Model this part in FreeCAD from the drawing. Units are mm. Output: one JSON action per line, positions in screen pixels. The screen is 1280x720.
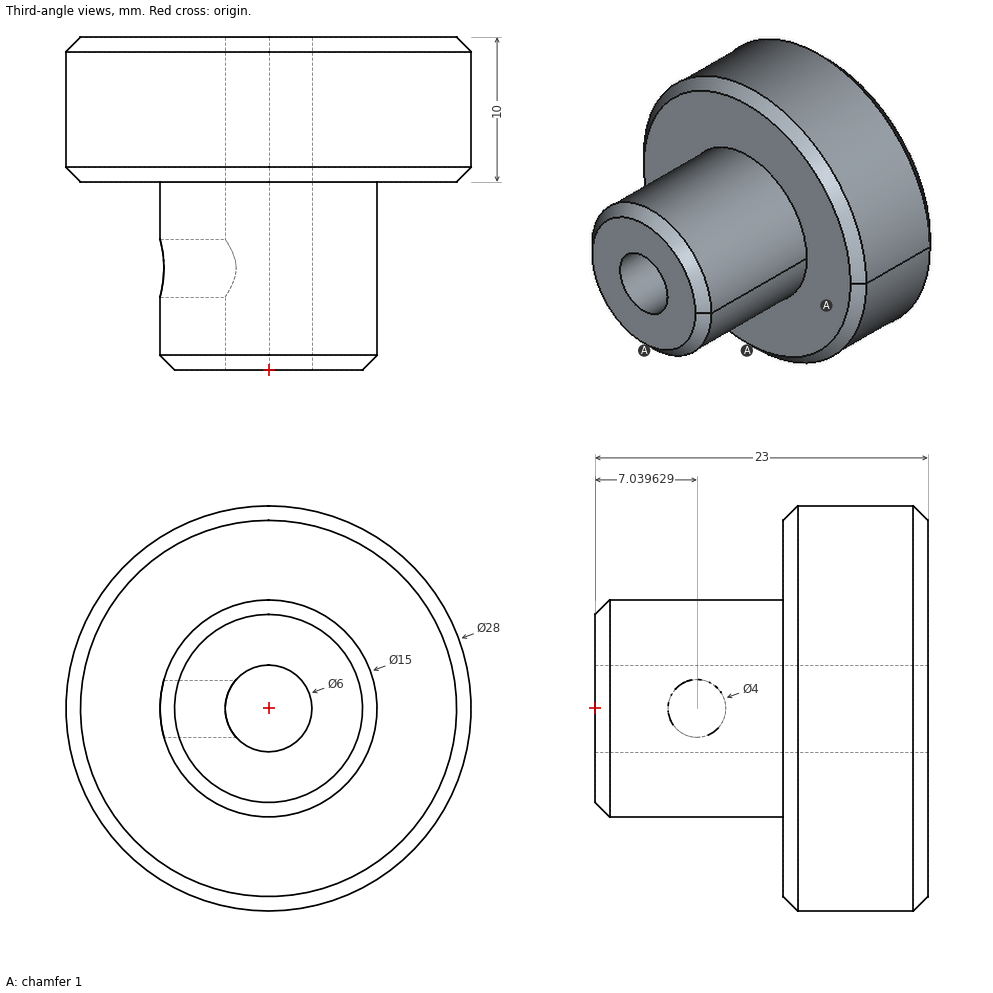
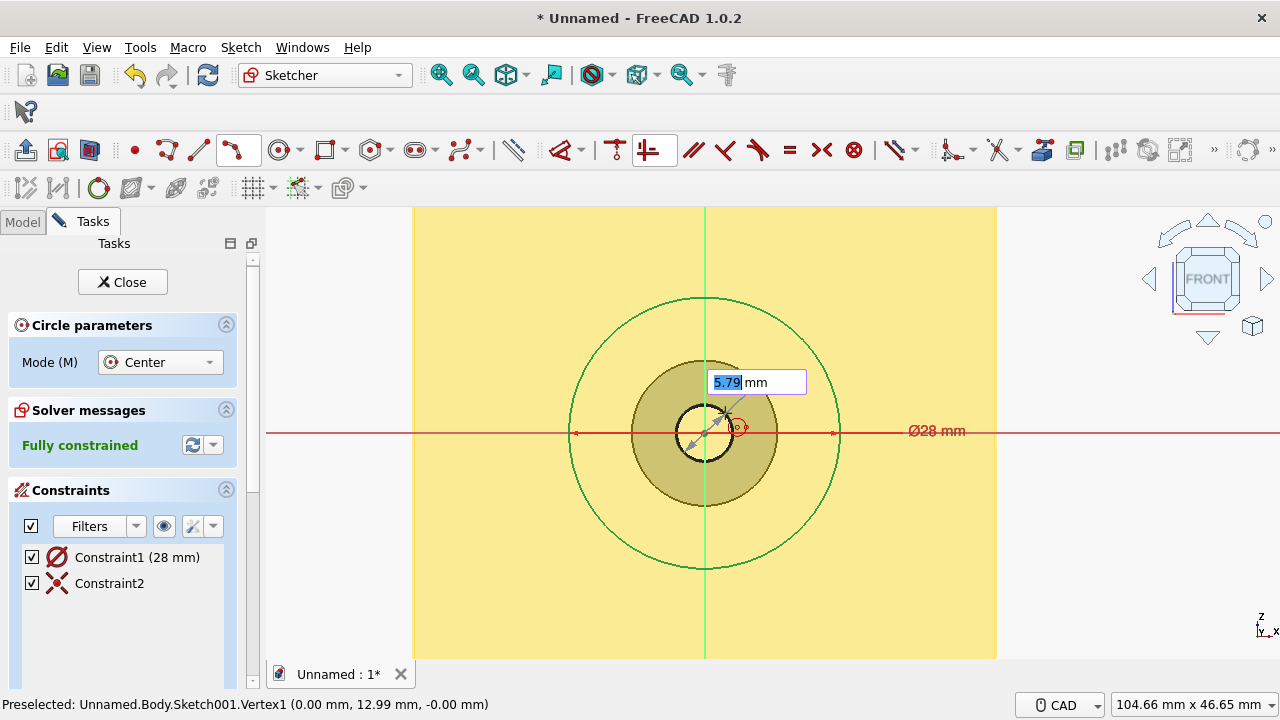
{"action": "type", "text": "6"}
{"action": "key", "text": "Return"}
{"action": "key", "text": "Escape"}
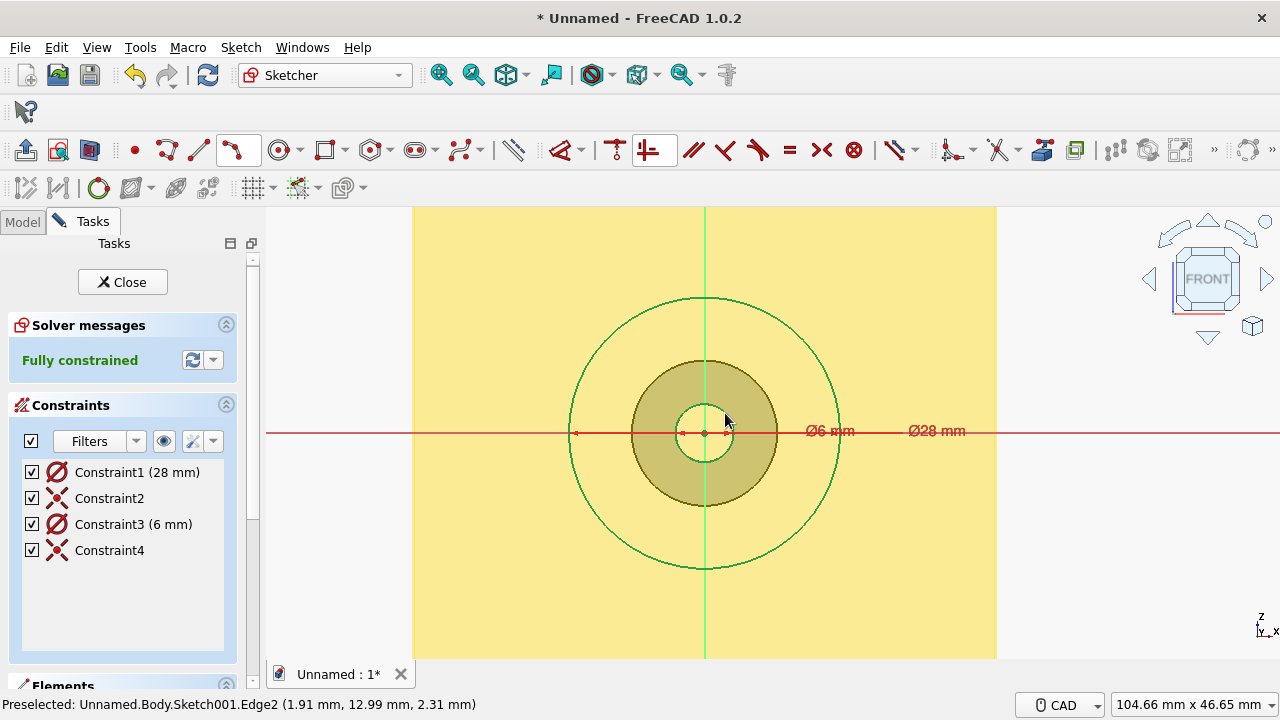
{"action": "left_click", "coordinate": [123, 282]}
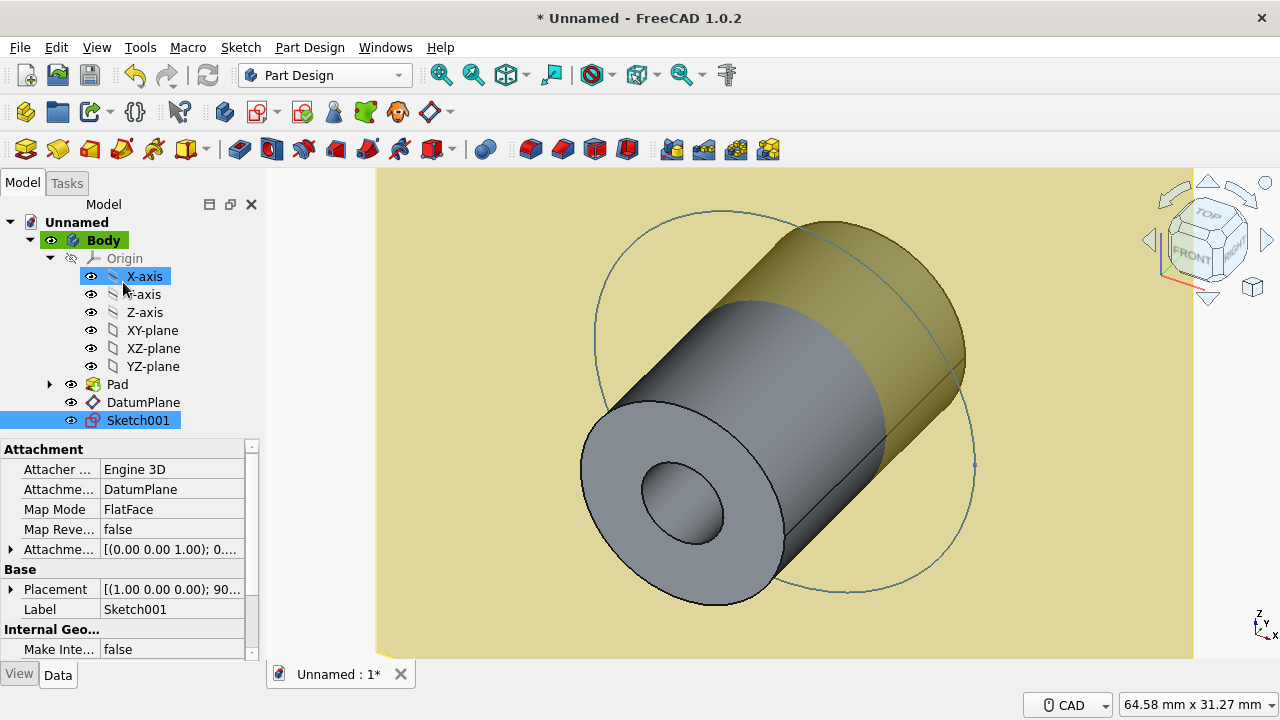
{"action": "left_click", "coordinate": [26, 150]}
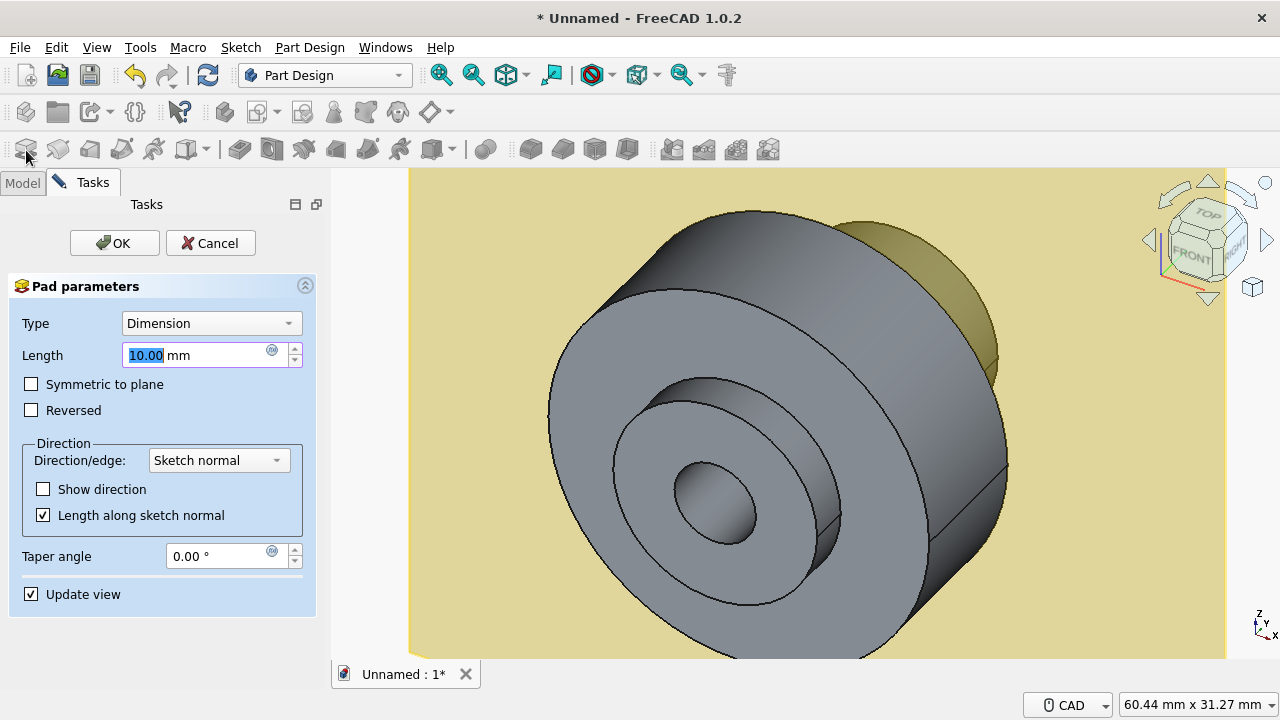
{"action": "type", "text": "10"}
{"action": "key", "text": "Tab"}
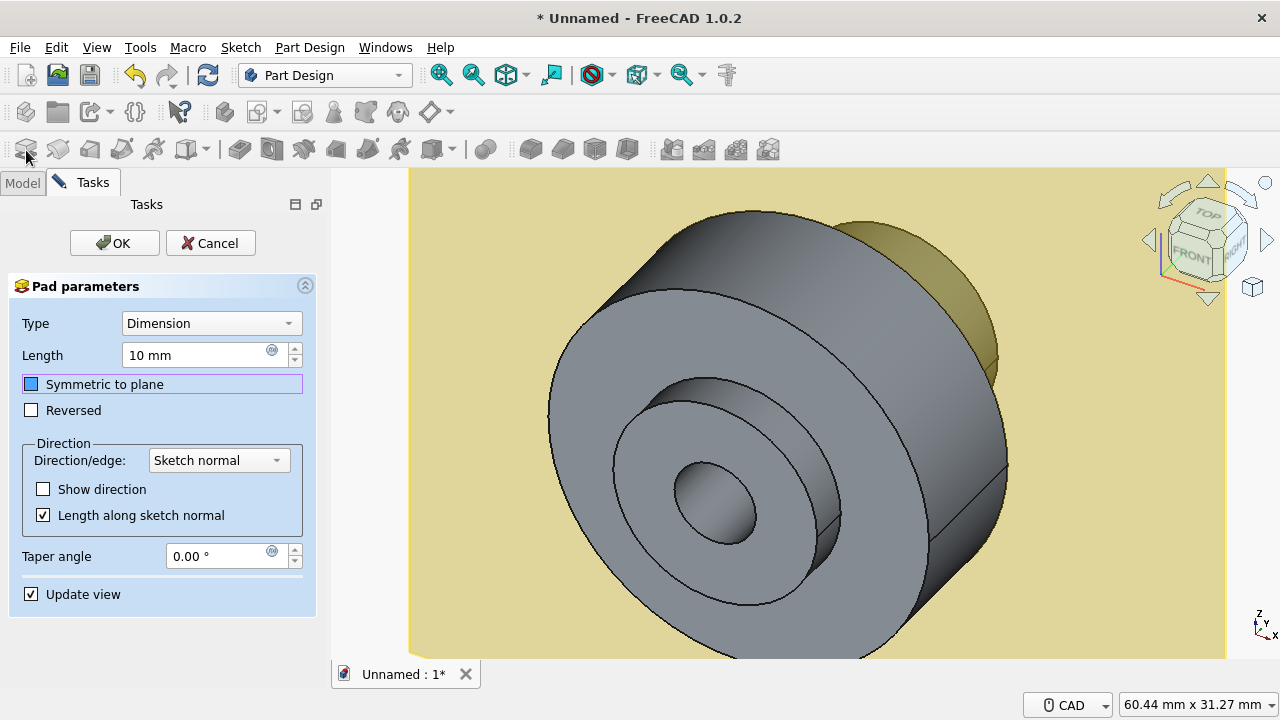
{"action": "left_click", "coordinate": [30, 410]}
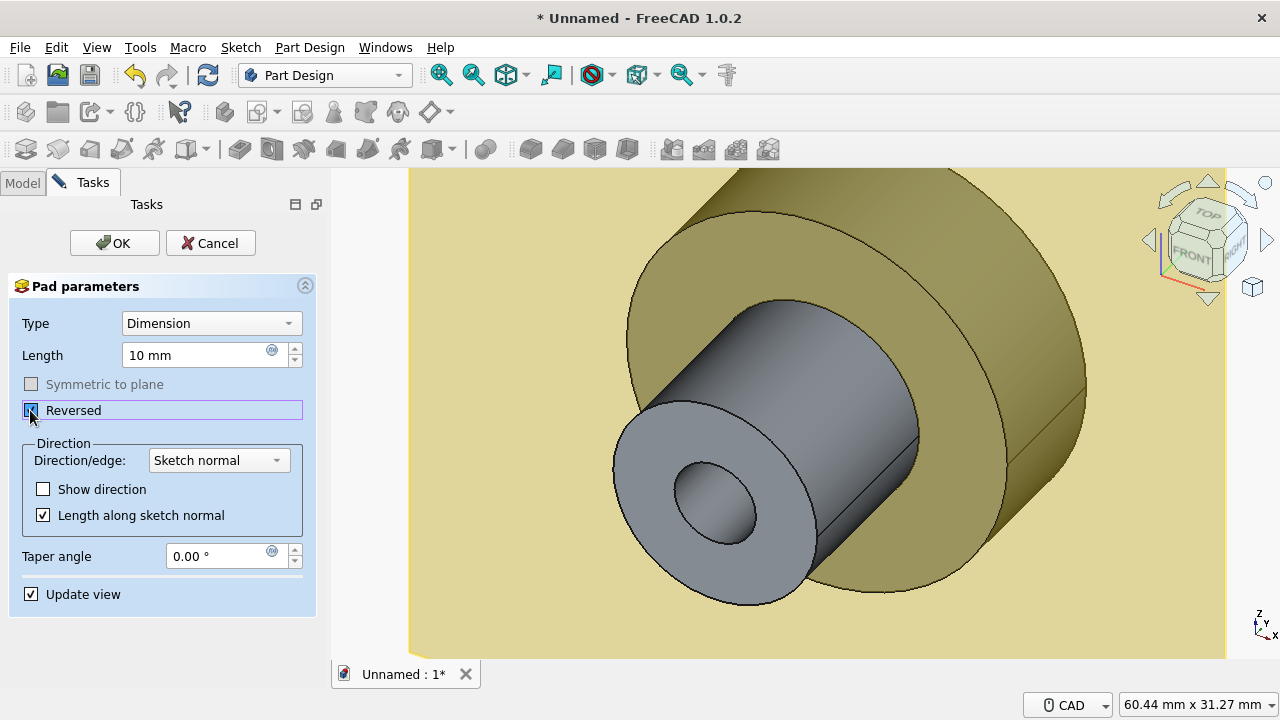
{"action": "left_click", "coordinate": [115, 243]}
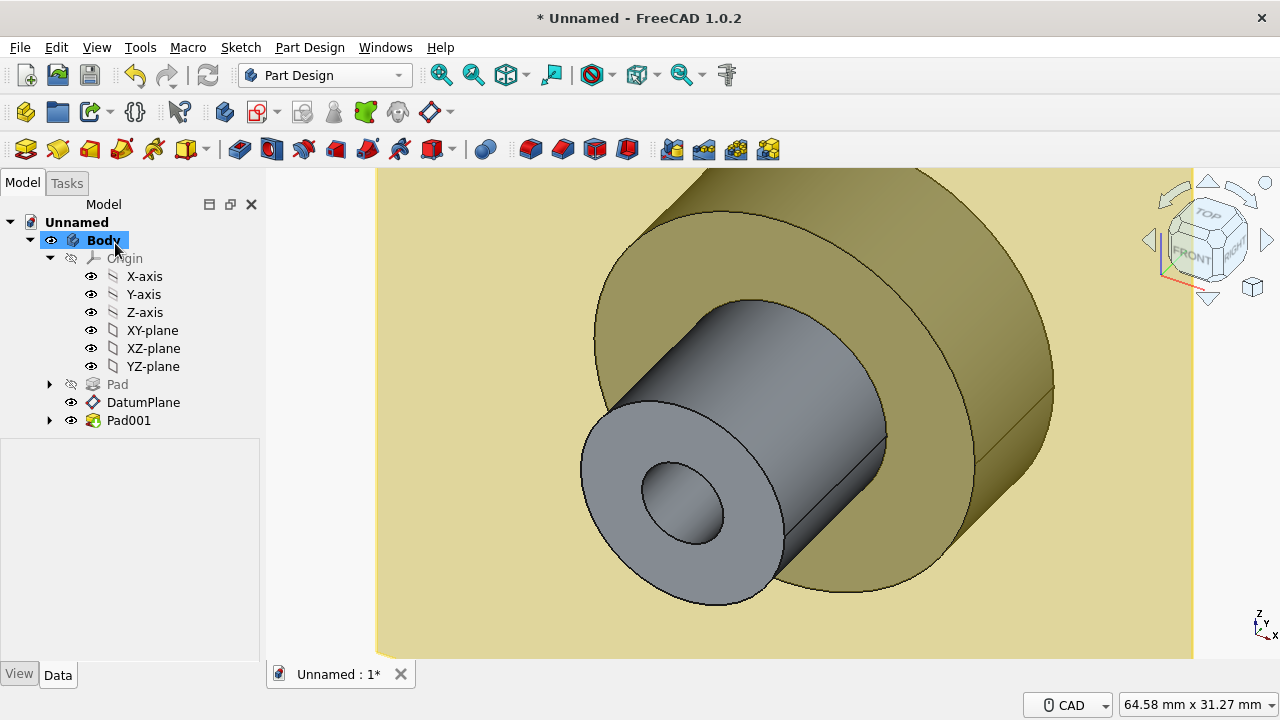
{"action": "left_click", "coordinate": [116, 402]}
{"action": "key", "text": "space"}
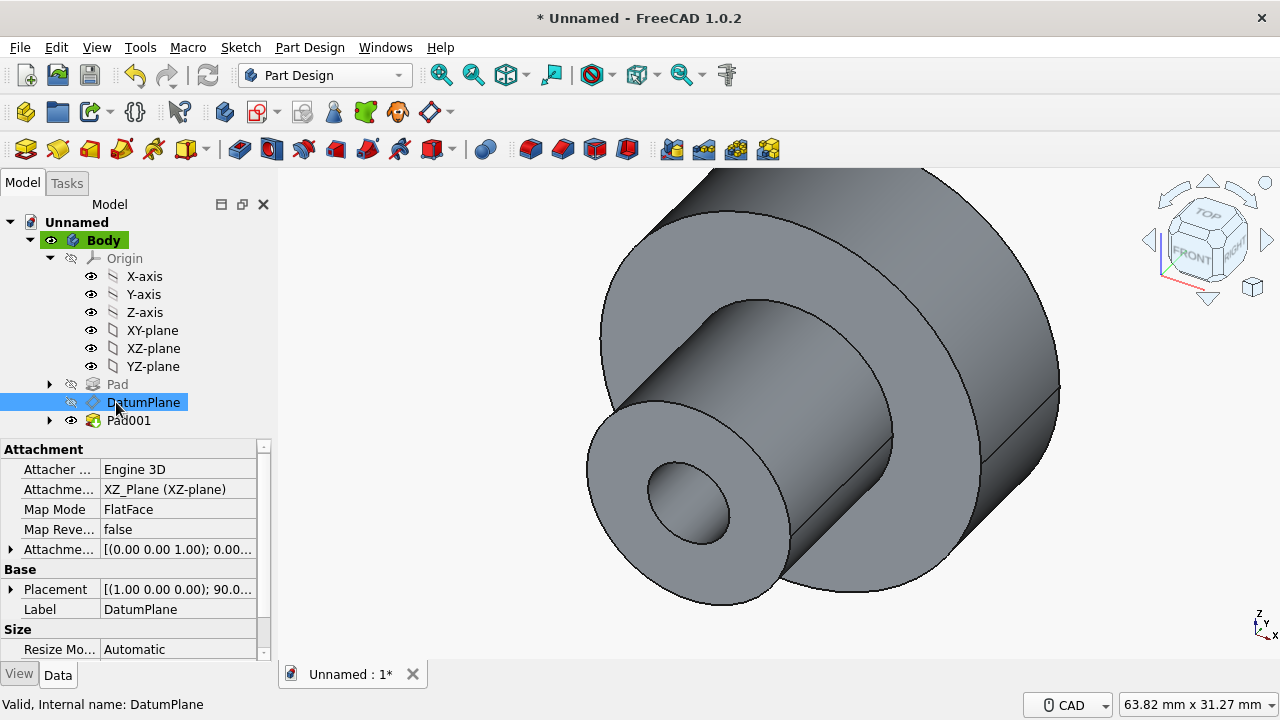
{"action": "left_click", "coordinate": [442, 76]}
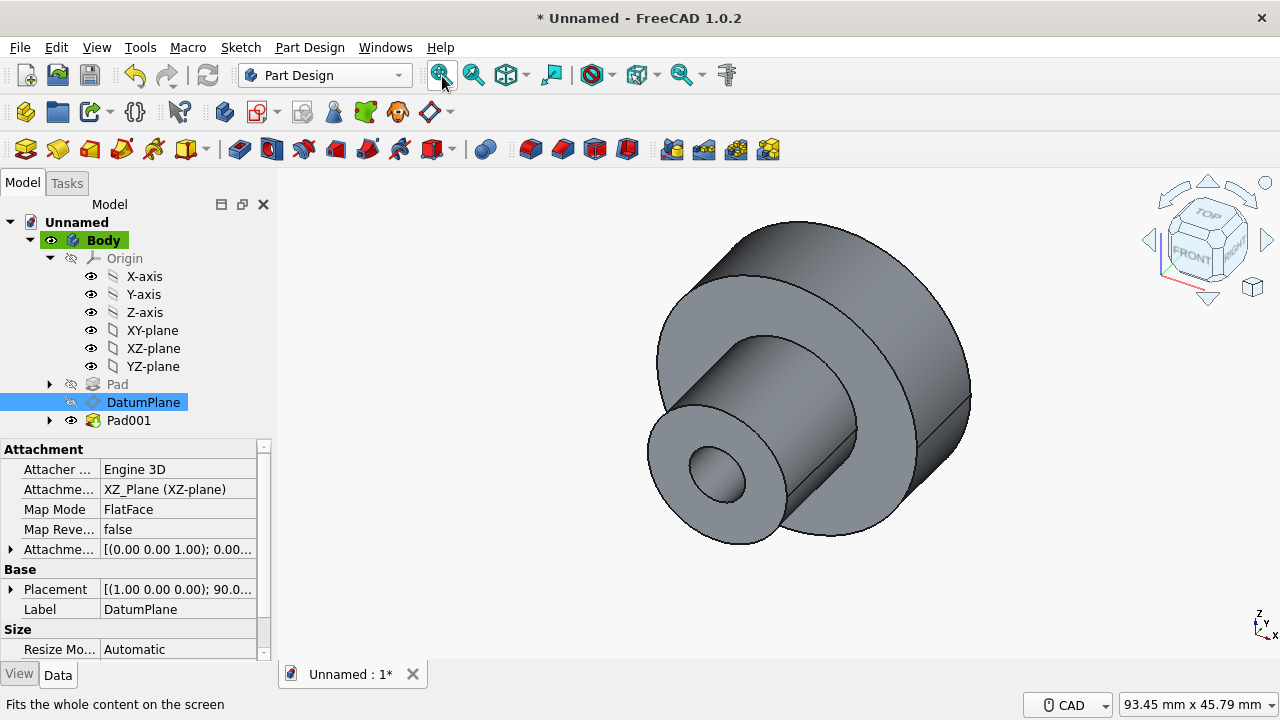
{"action": "left_click", "coordinate": [682, 297]}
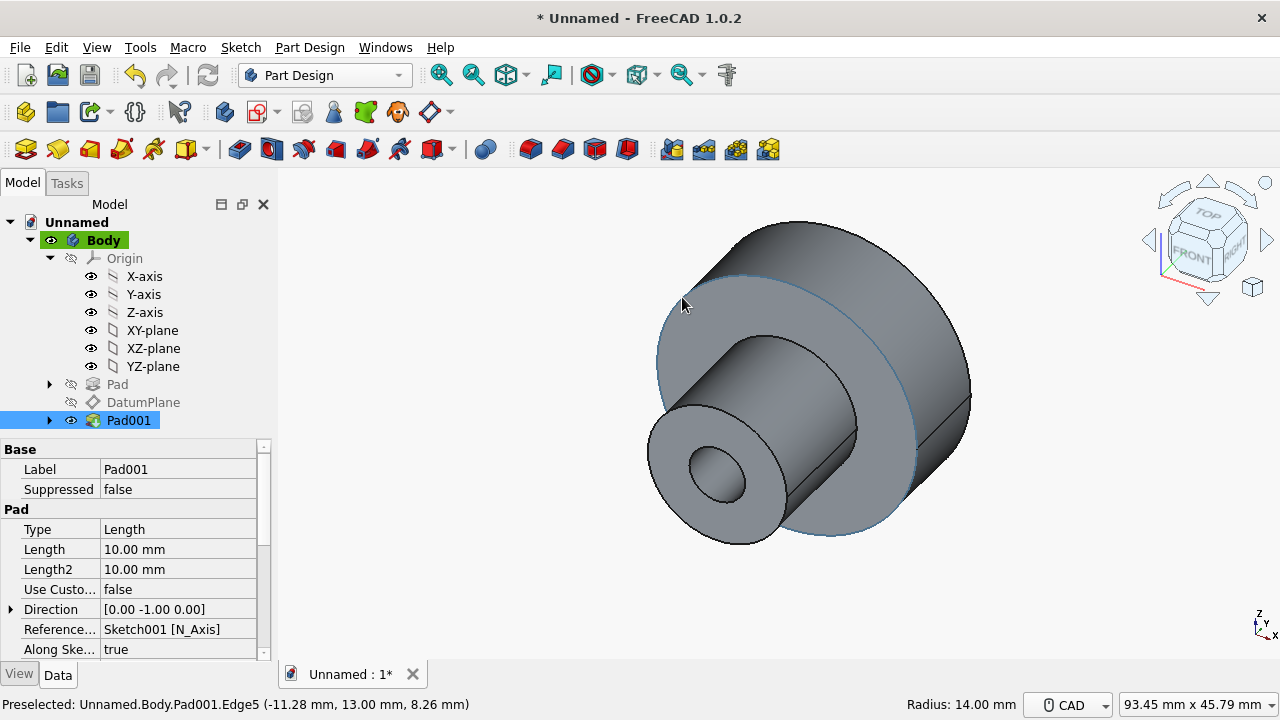
{"action": "left_click", "coordinate": [661, 416], "text": "ctrl"}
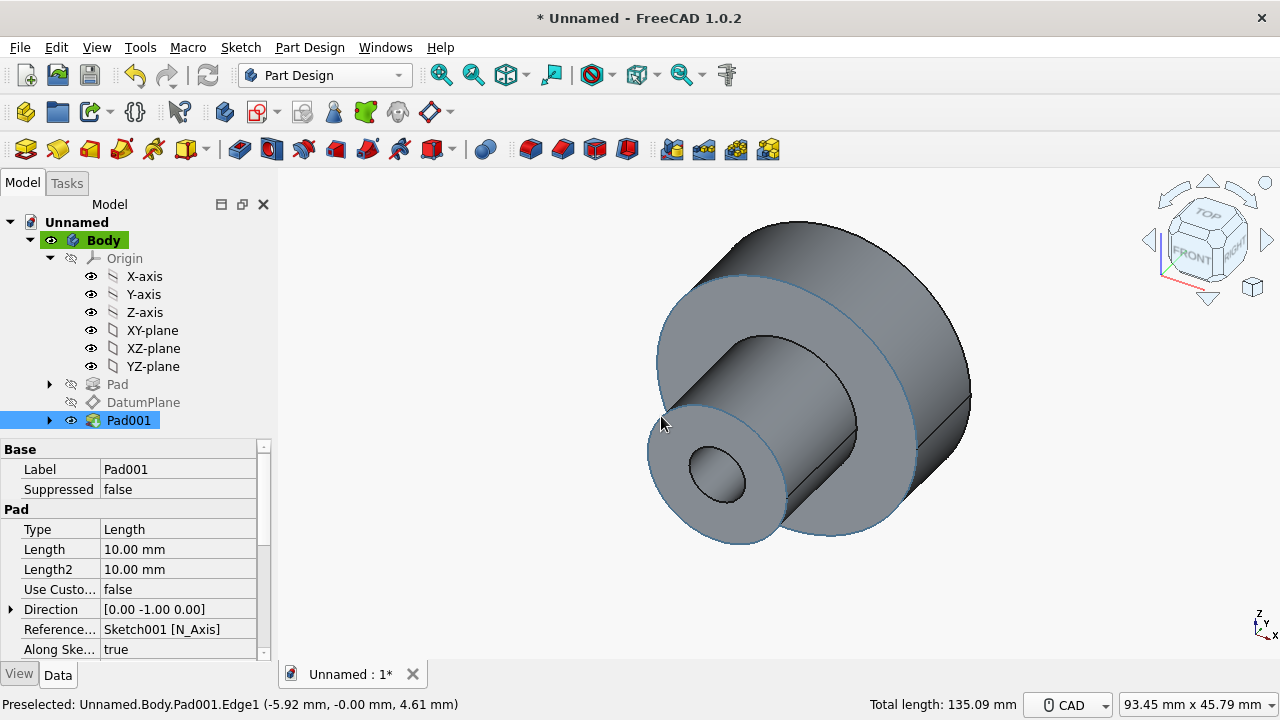
{"action": "key", "text": "0"}